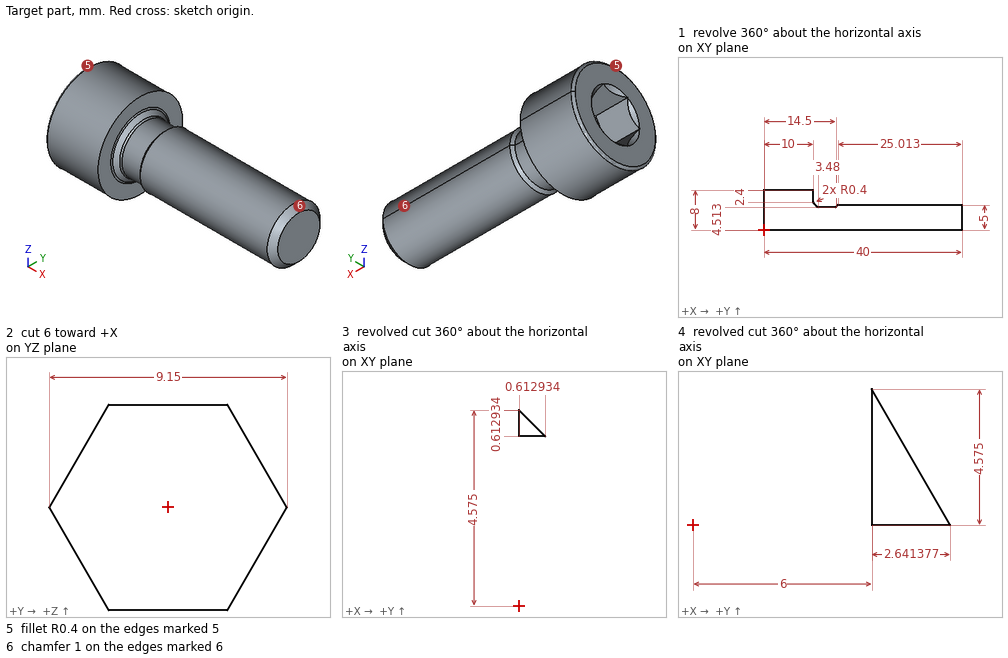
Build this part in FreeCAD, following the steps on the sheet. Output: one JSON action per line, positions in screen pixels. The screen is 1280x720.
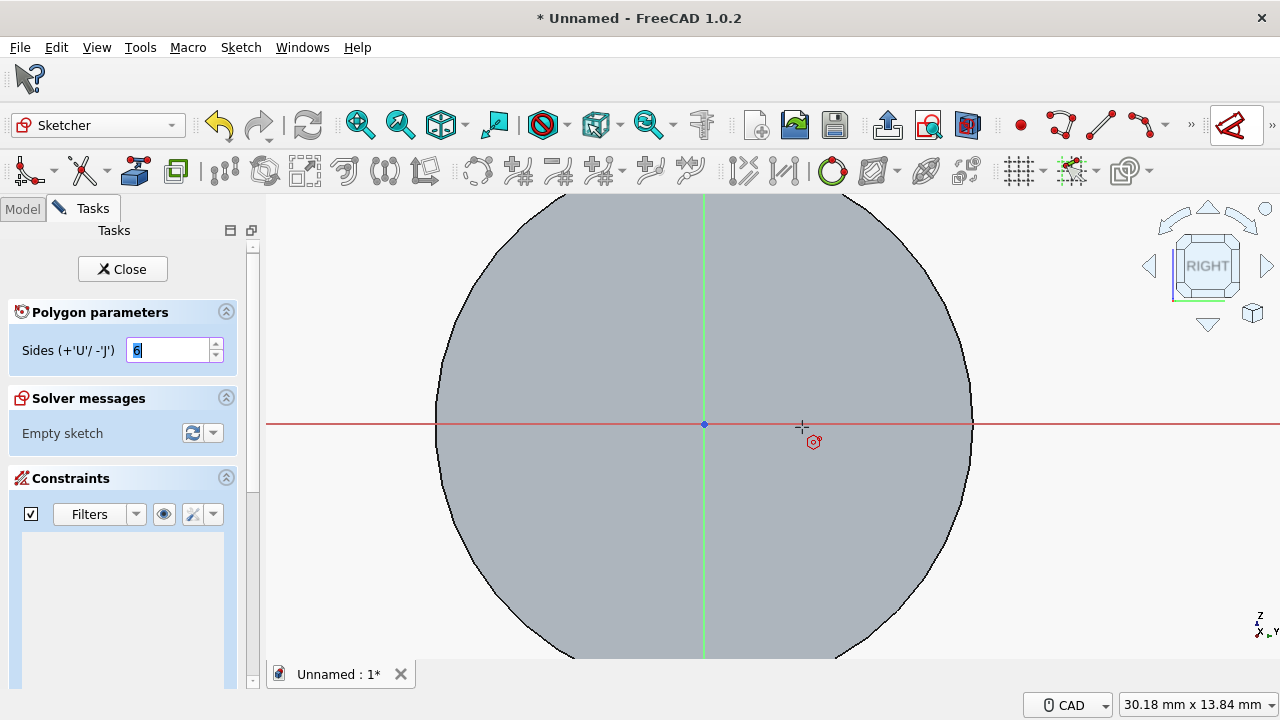
{"action": "left_click", "coordinate": [704, 424]}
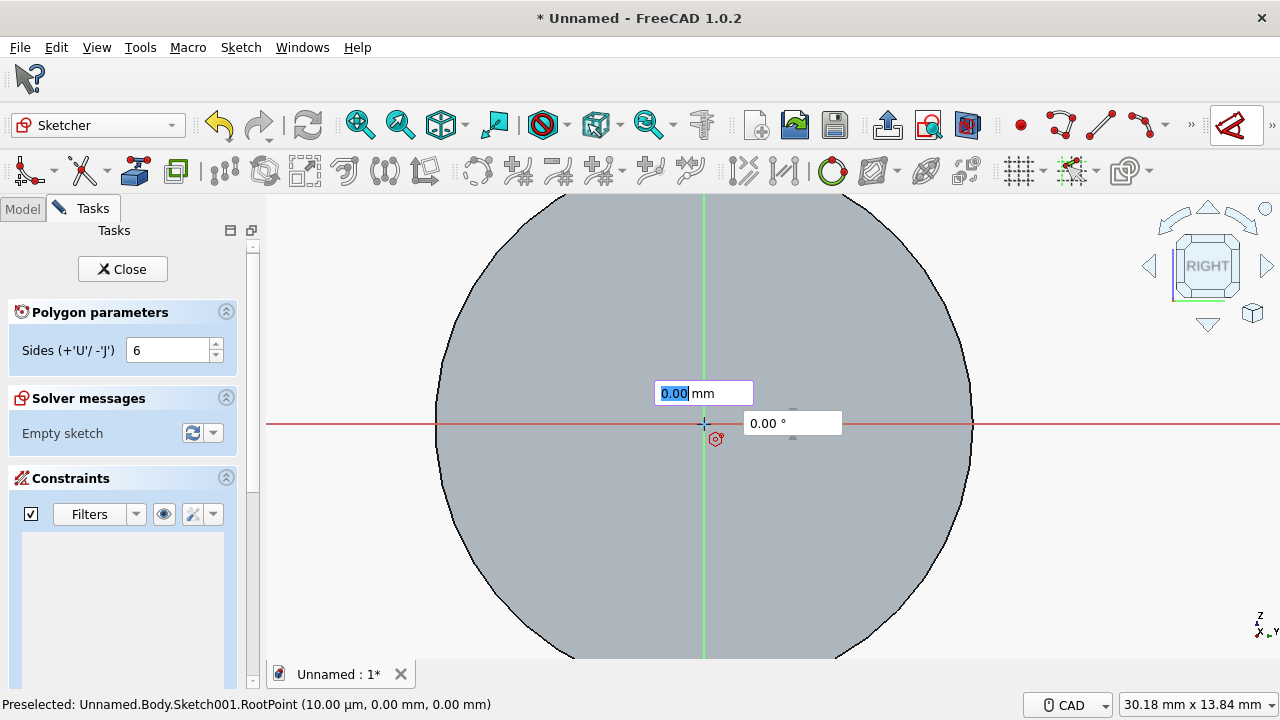
{"action": "left_click", "coordinate": [858, 424]}
{"action": "key", "text": "Escape"}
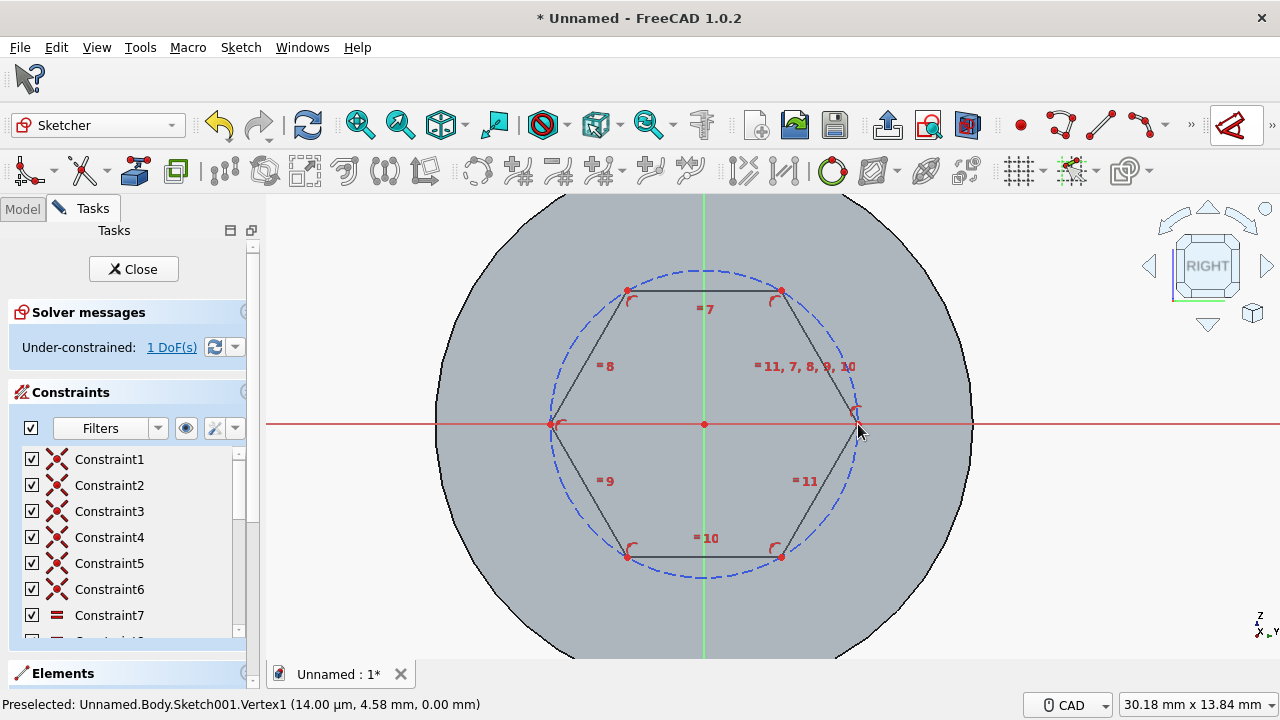
{"action": "left_click", "coordinate": [550, 424]}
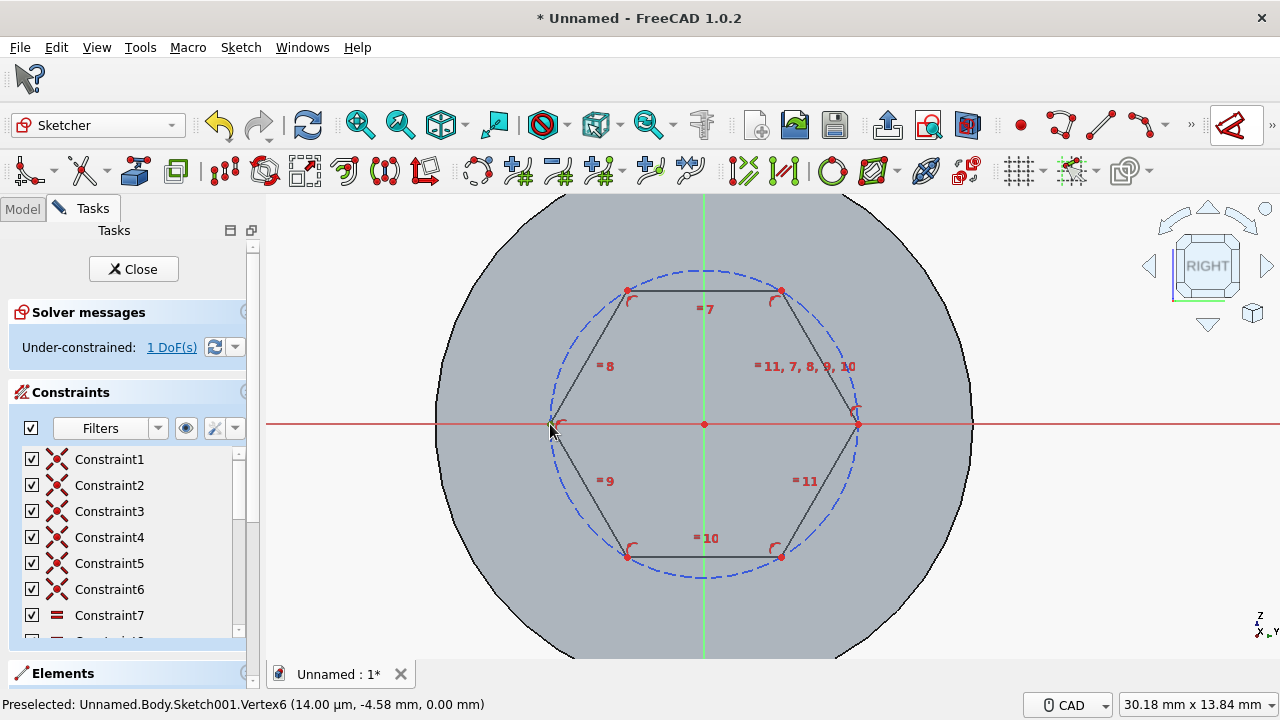
{"action": "left_click", "coordinate": [858, 424]}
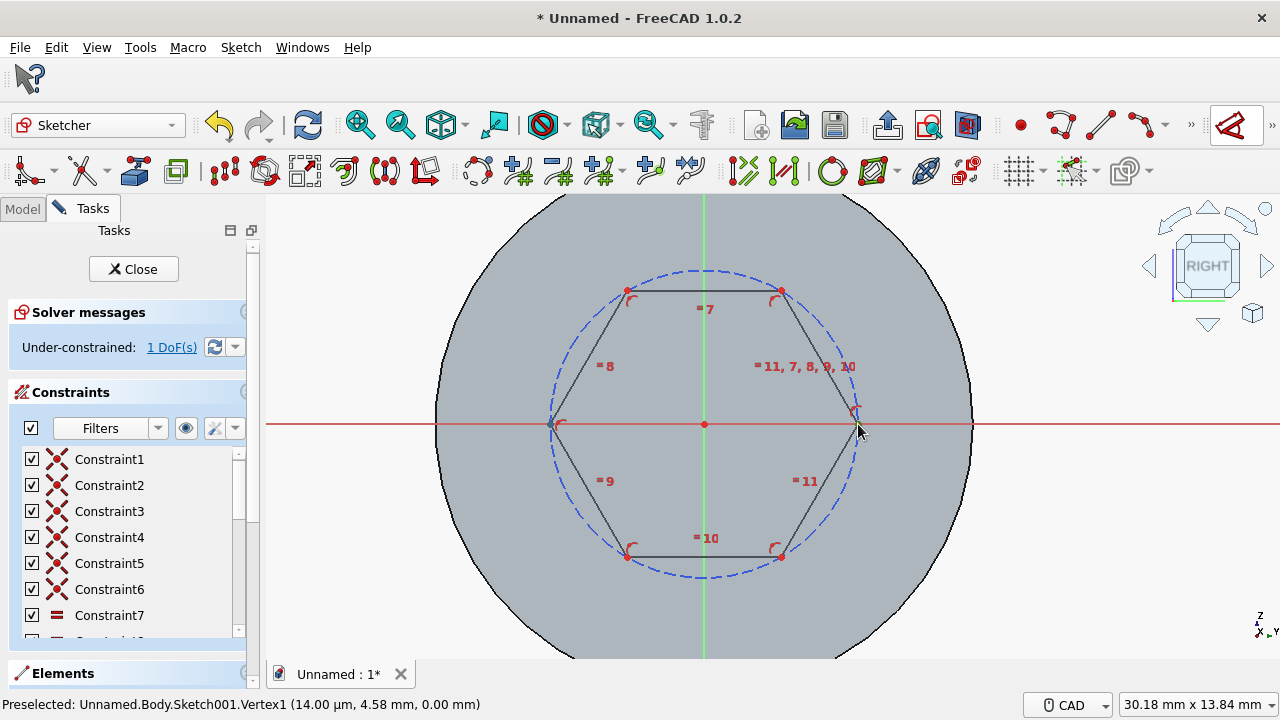
{"action": "left_click", "coordinate": [1258, 126]}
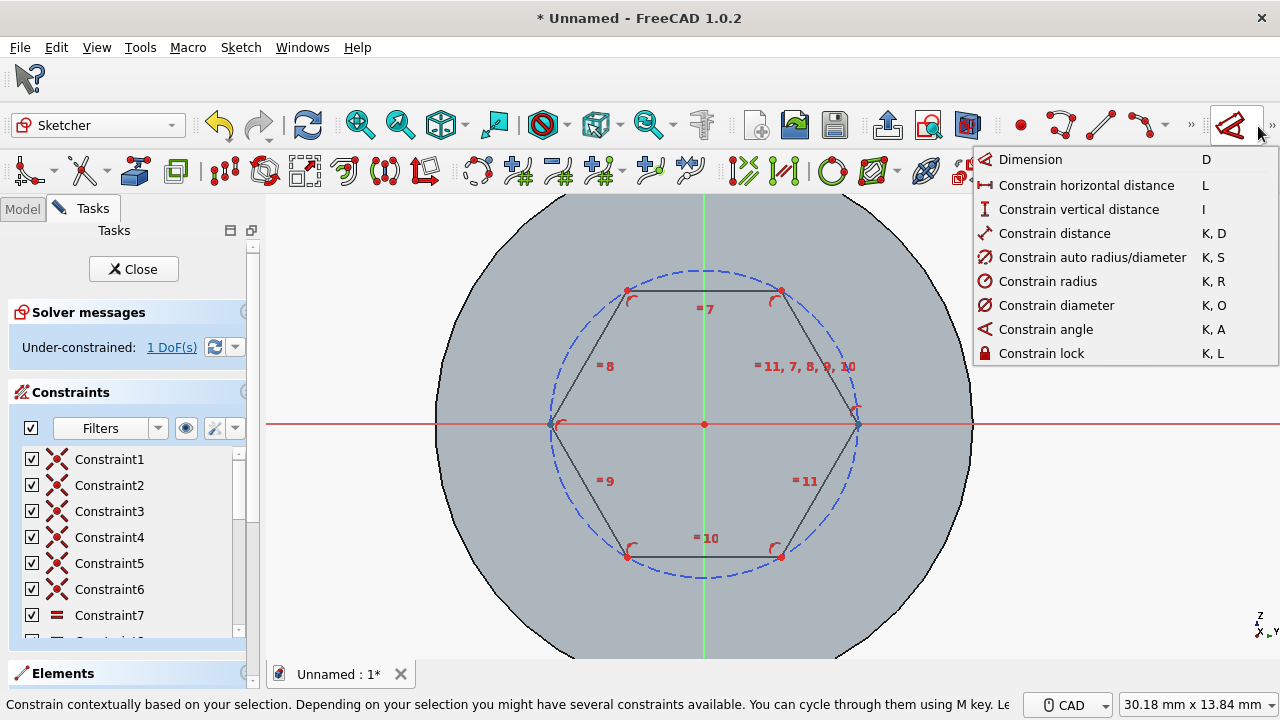
{"action": "left_click", "coordinate": [1126, 185]}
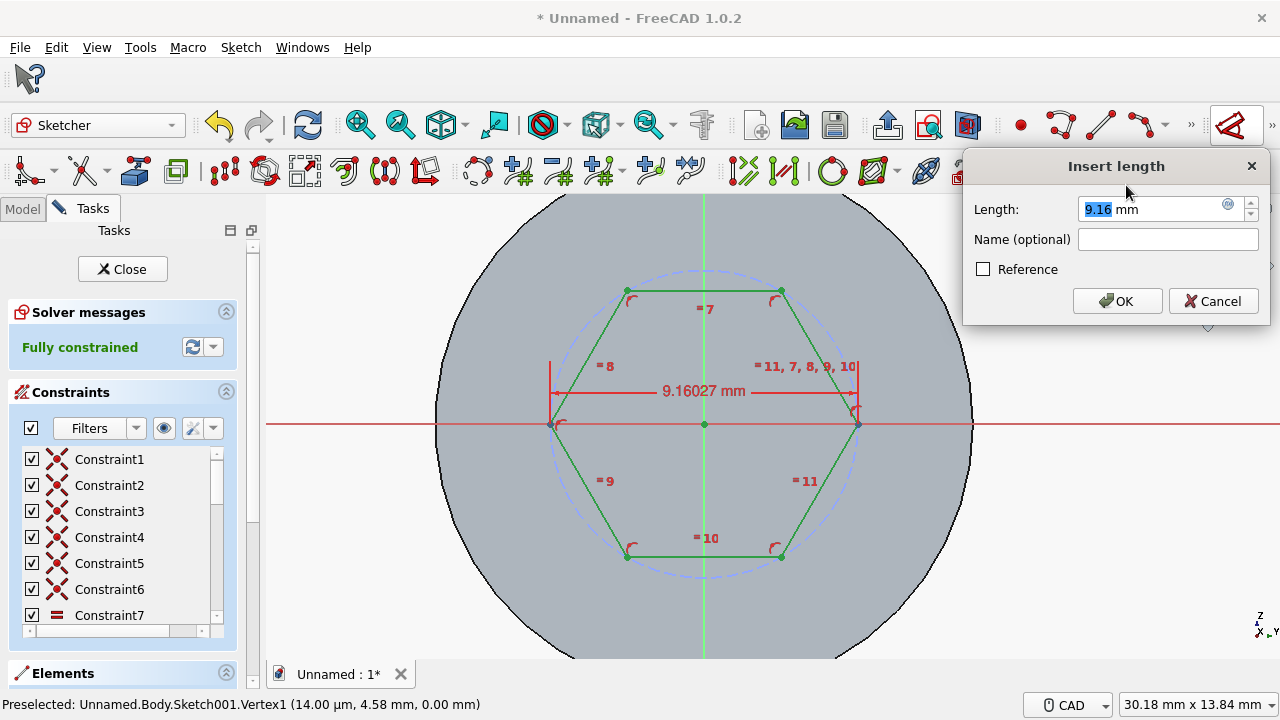
{"action": "type", "text": "9.15"}
{"action": "key", "text": "Return"}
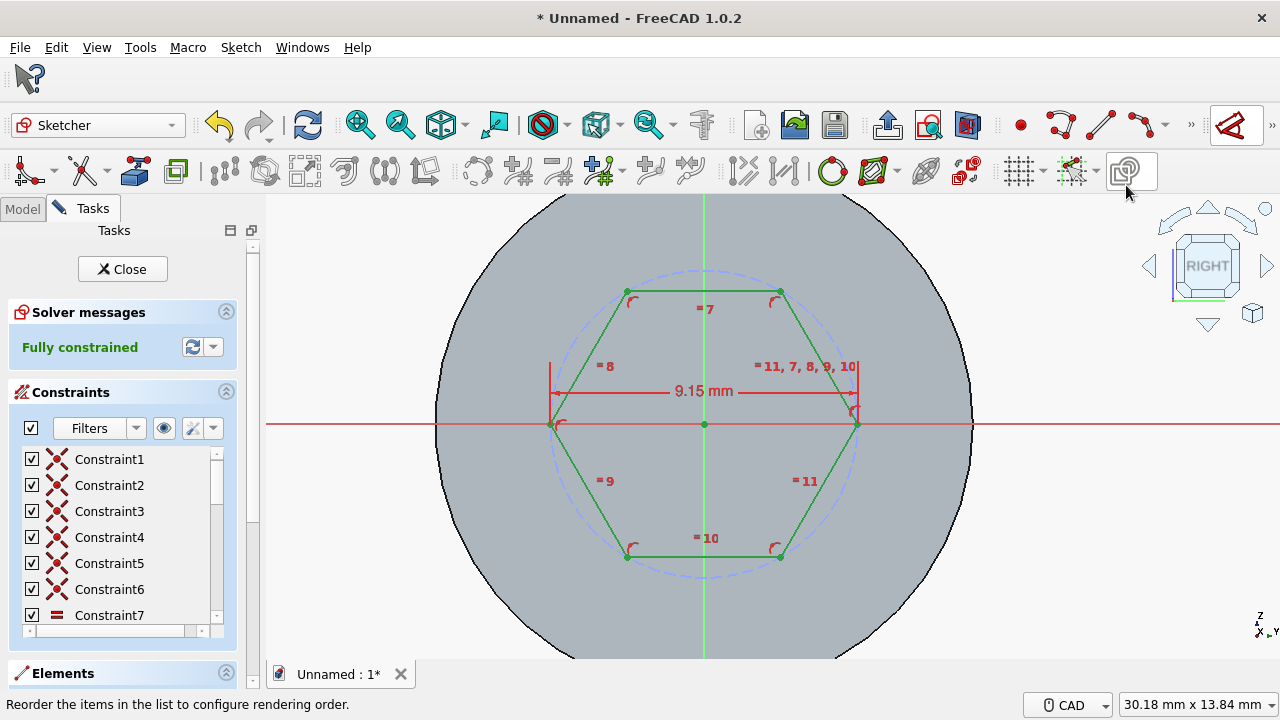
{"action": "left_click", "coordinate": [123, 269]}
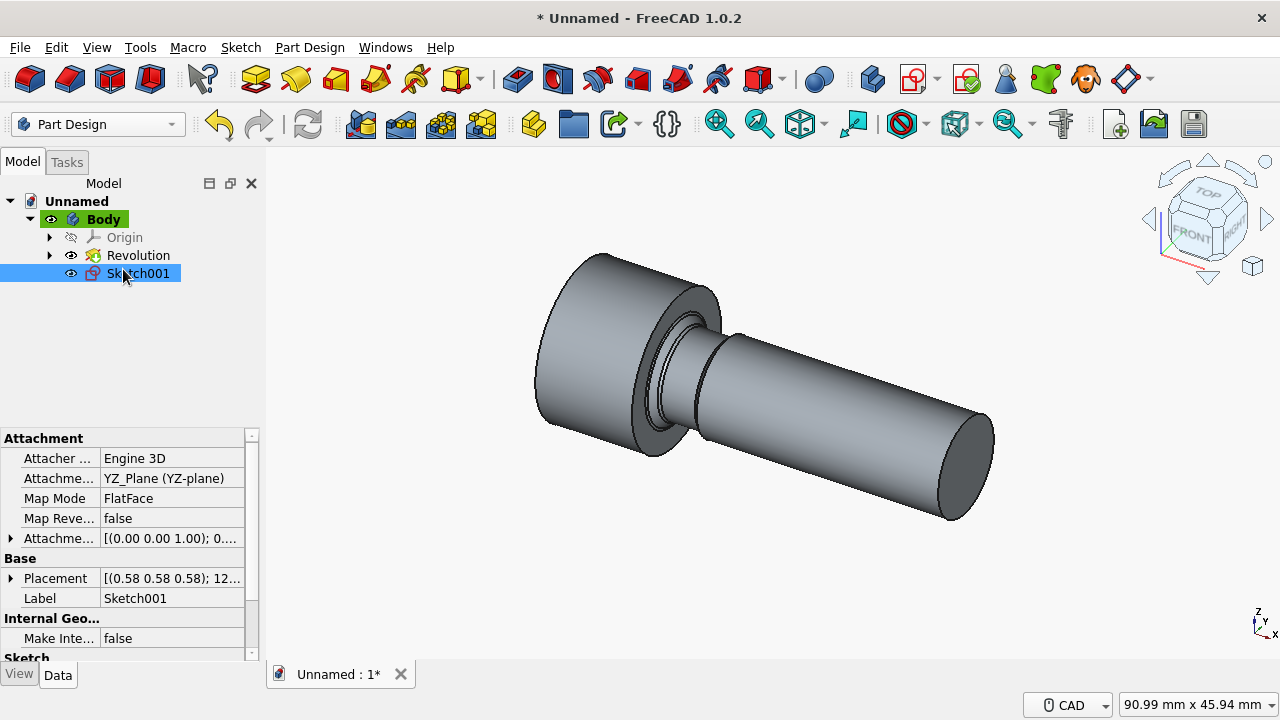
{"action": "left_click", "coordinate": [518, 80]}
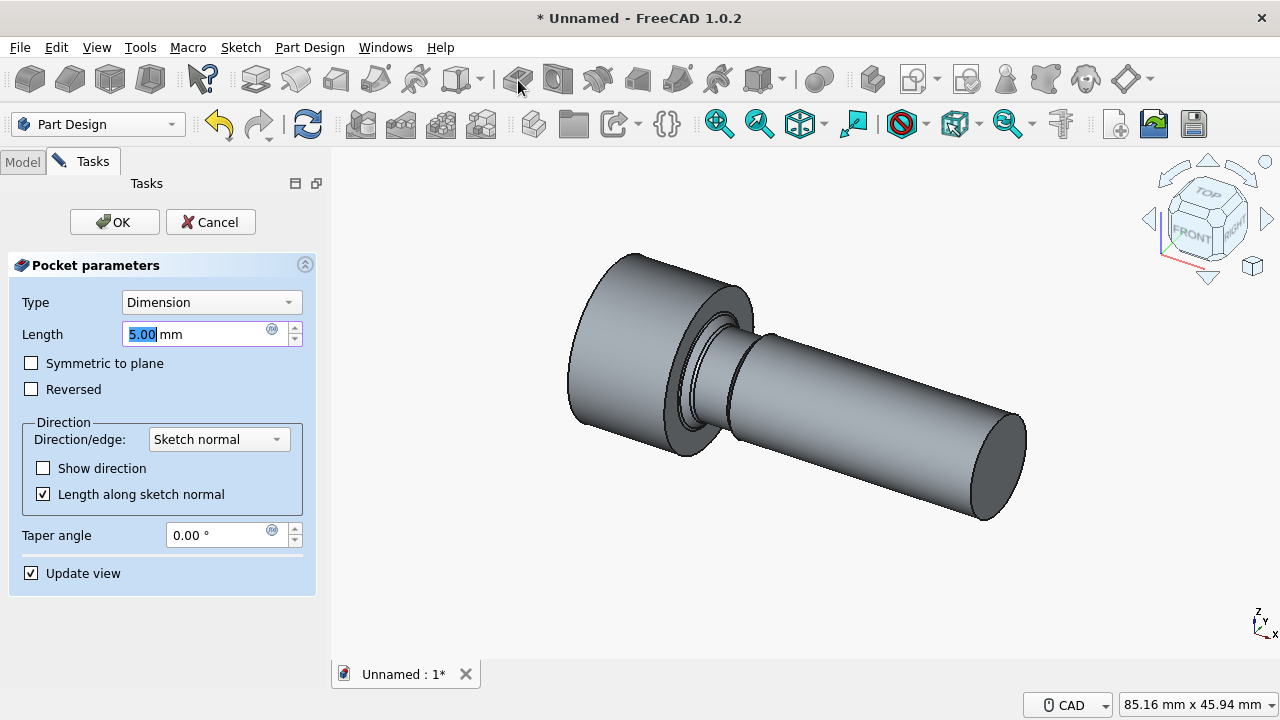
{"action": "type", "text": "6"}
{"action": "key", "text": "Tab"}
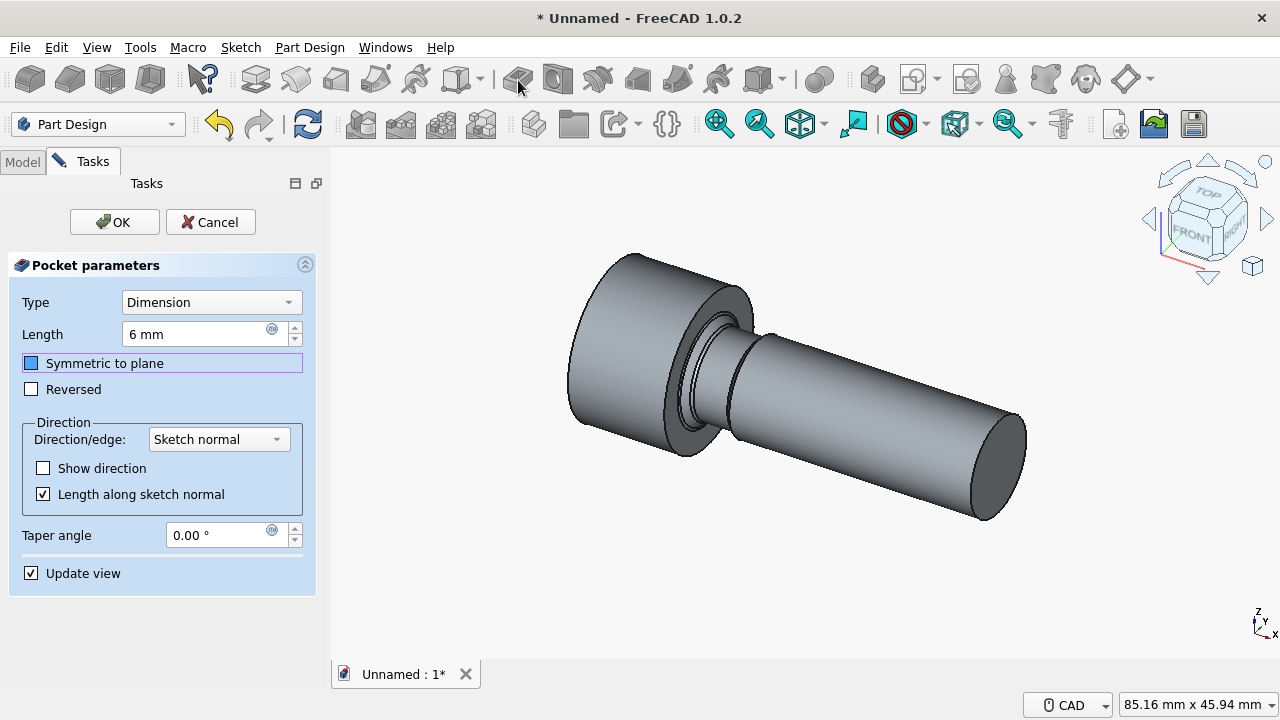
{"action": "left_click", "coordinate": [30, 389]}